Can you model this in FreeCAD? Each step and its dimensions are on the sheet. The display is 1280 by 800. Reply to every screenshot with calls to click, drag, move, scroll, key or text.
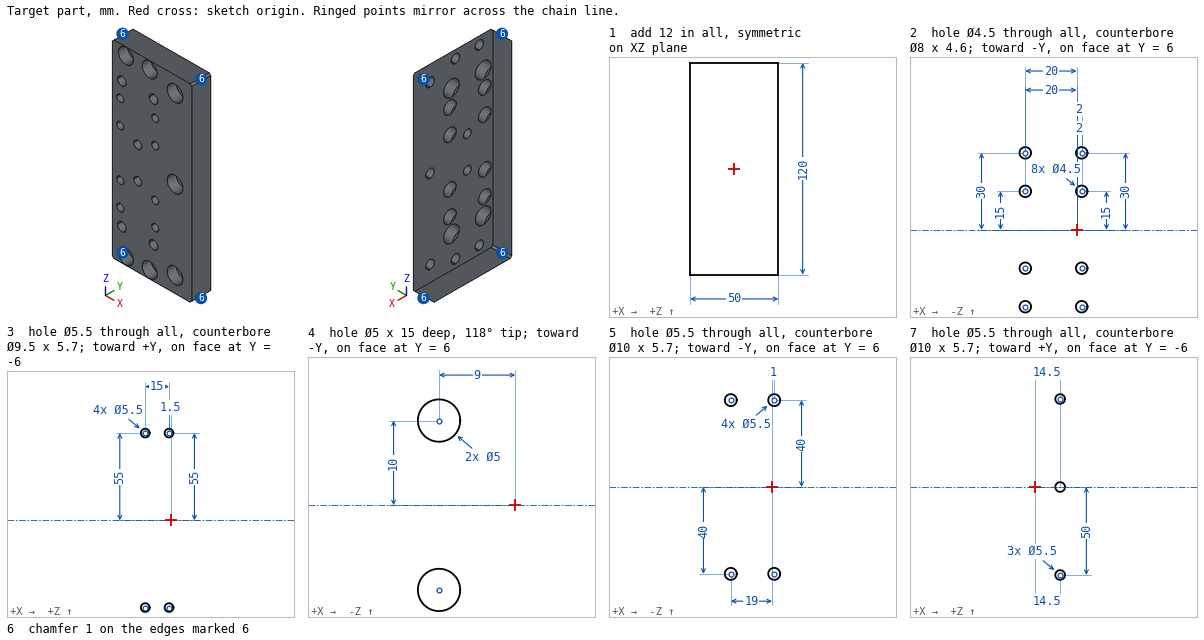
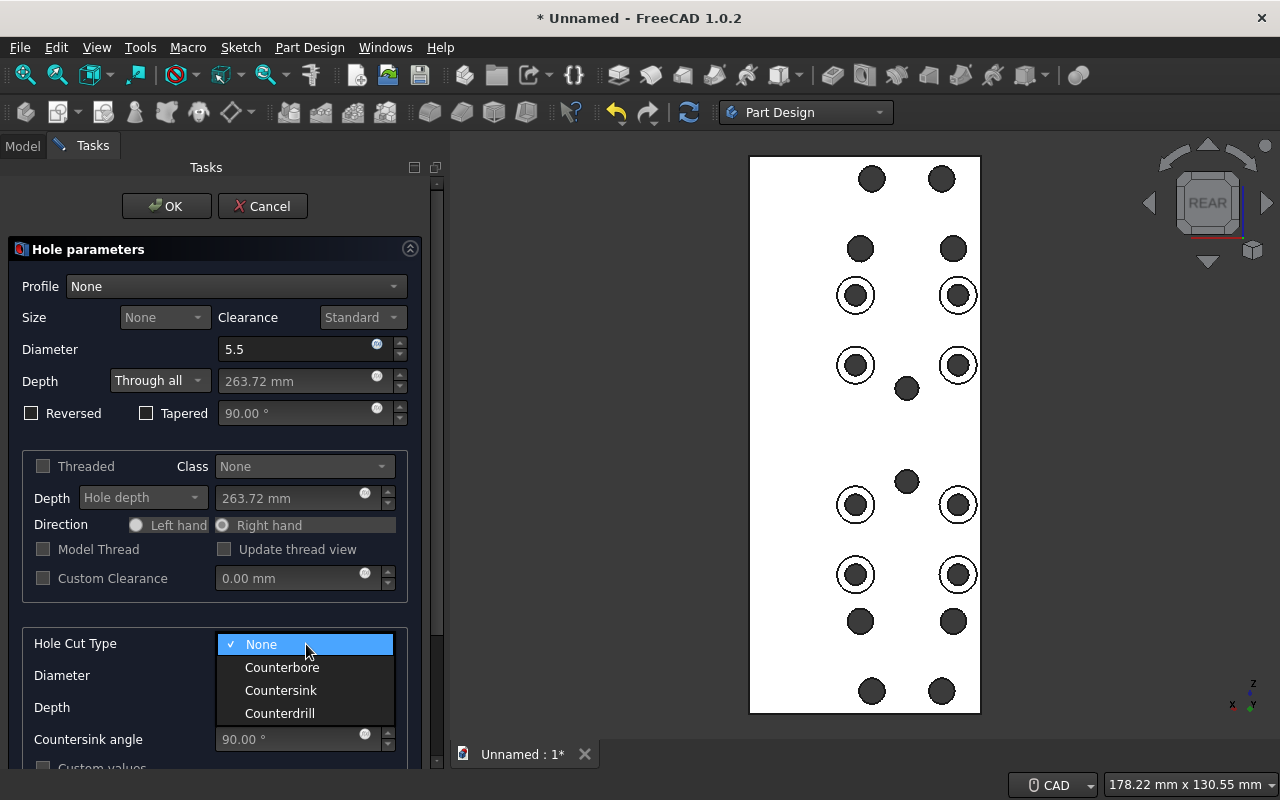
click(304, 668)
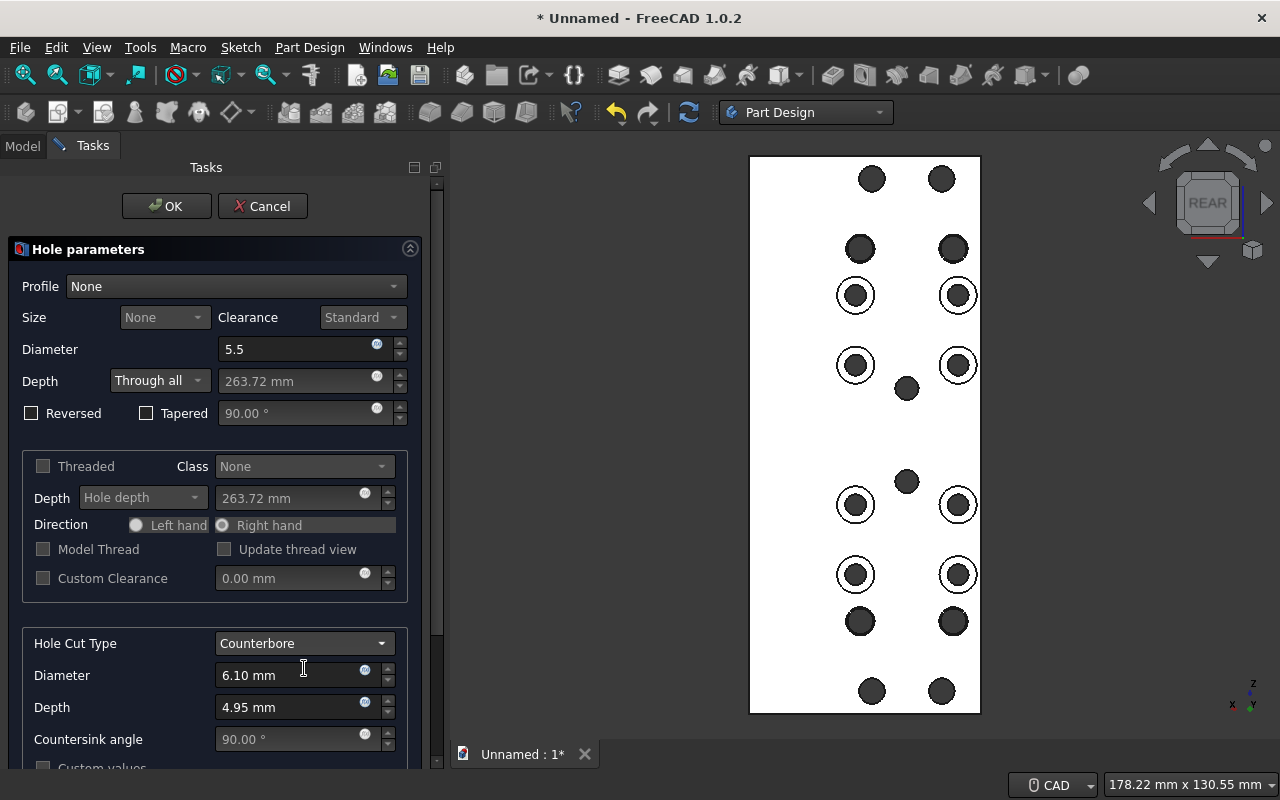
triple_click(298, 675)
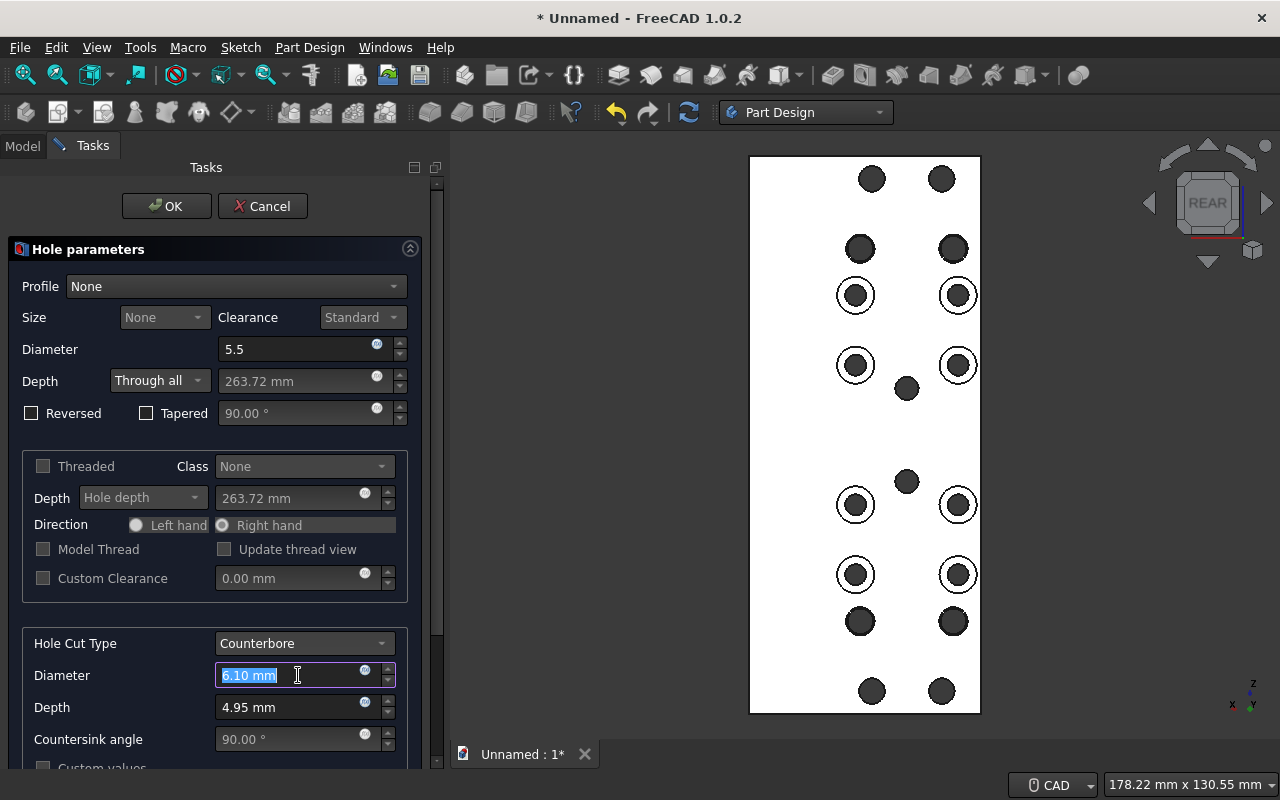
text(10)
key(Tab)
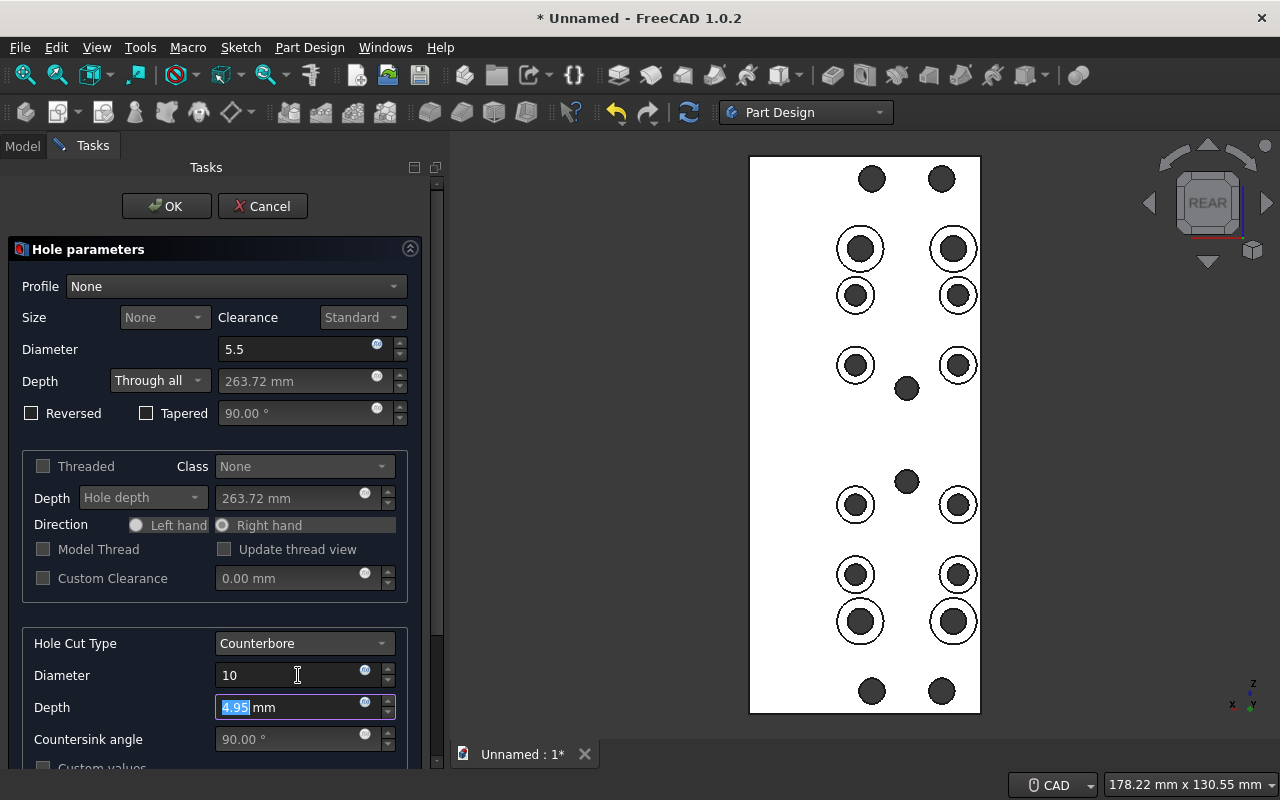
text(5.7)
key(Tab)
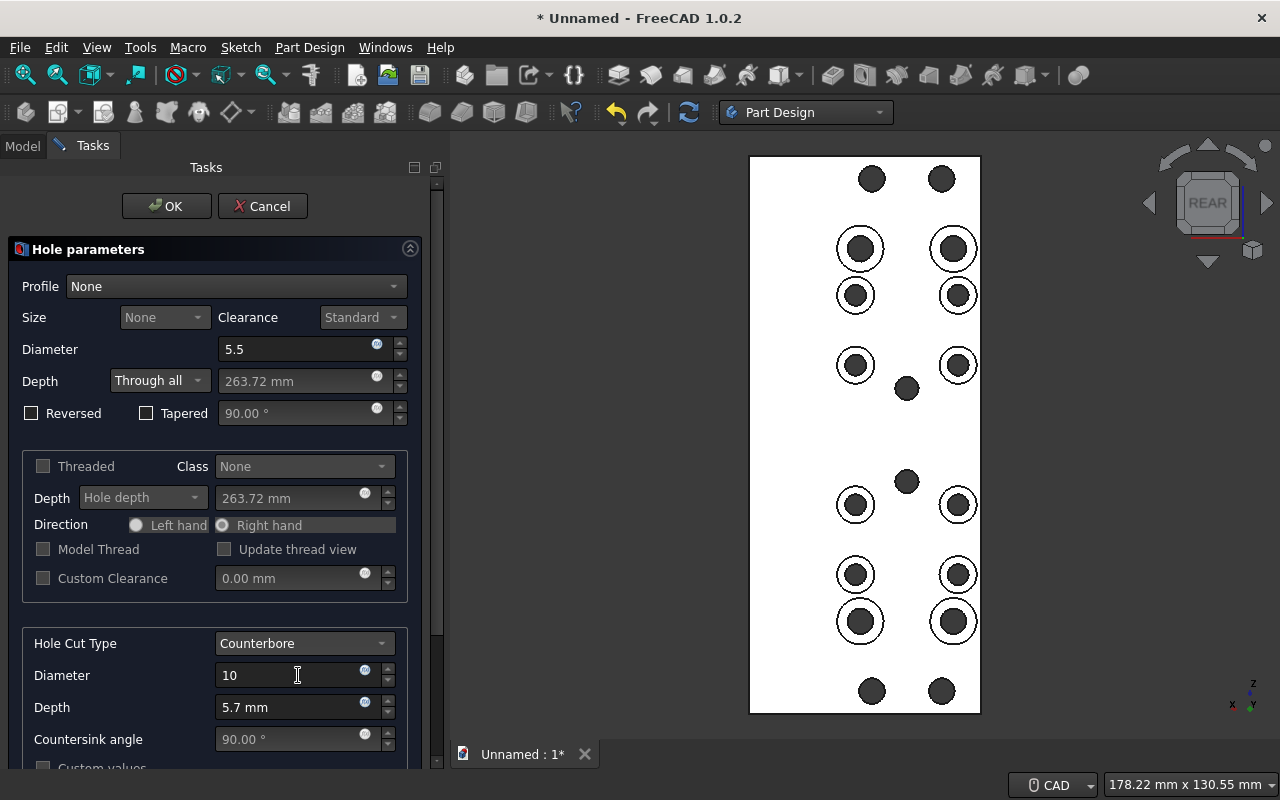
click(167, 206)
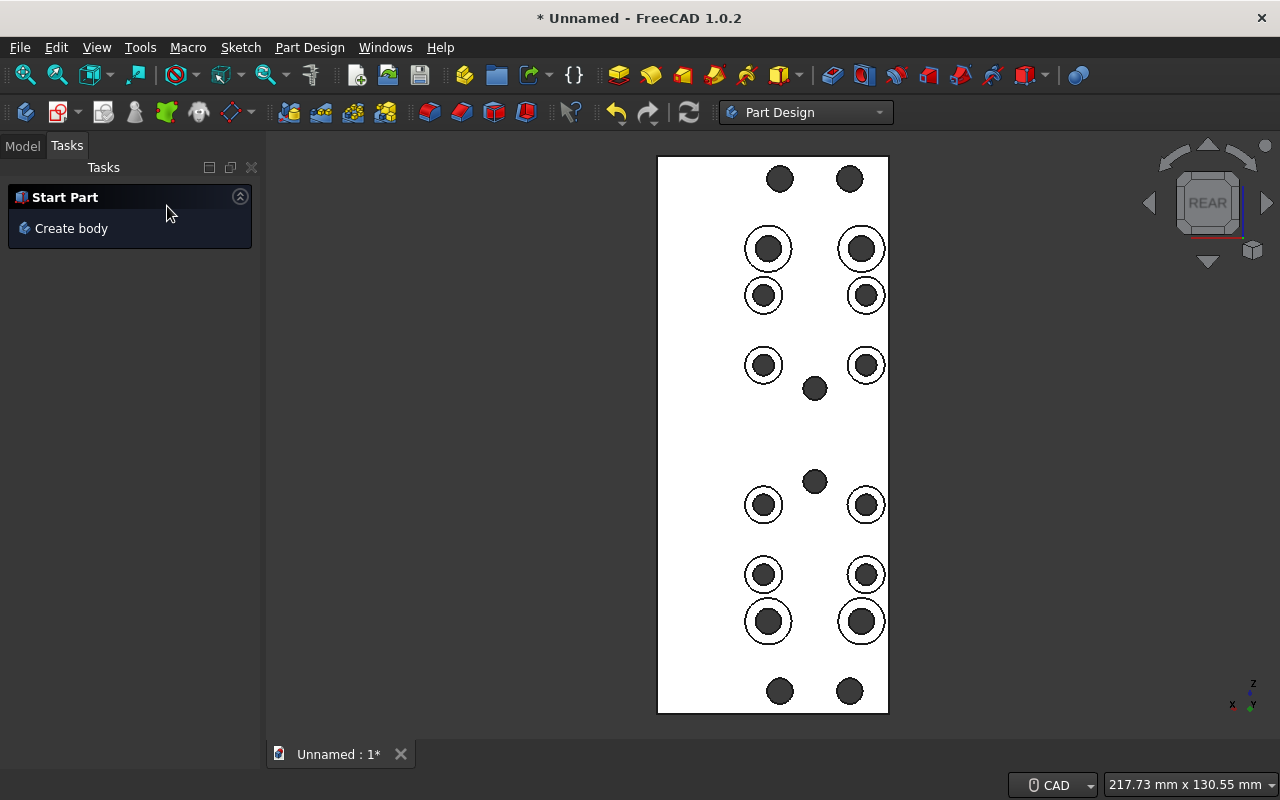
key(0)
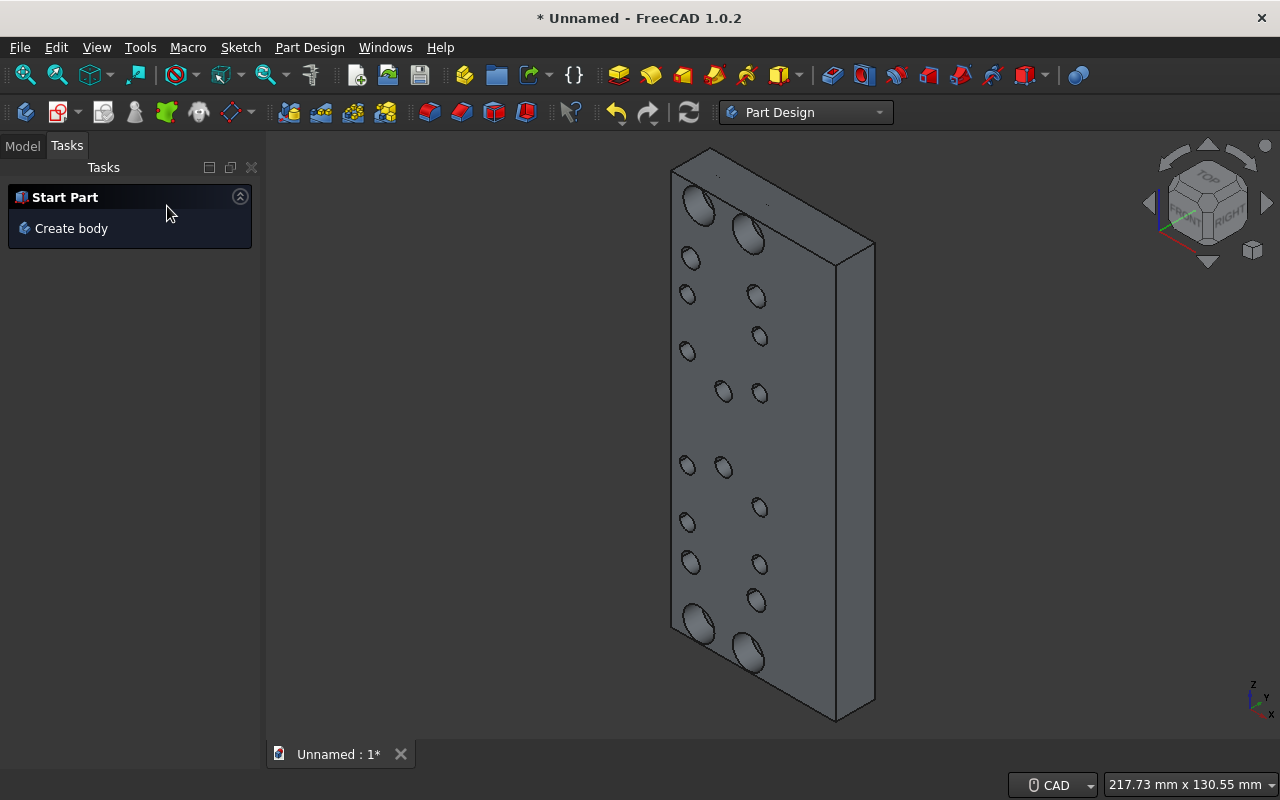
click(855, 253)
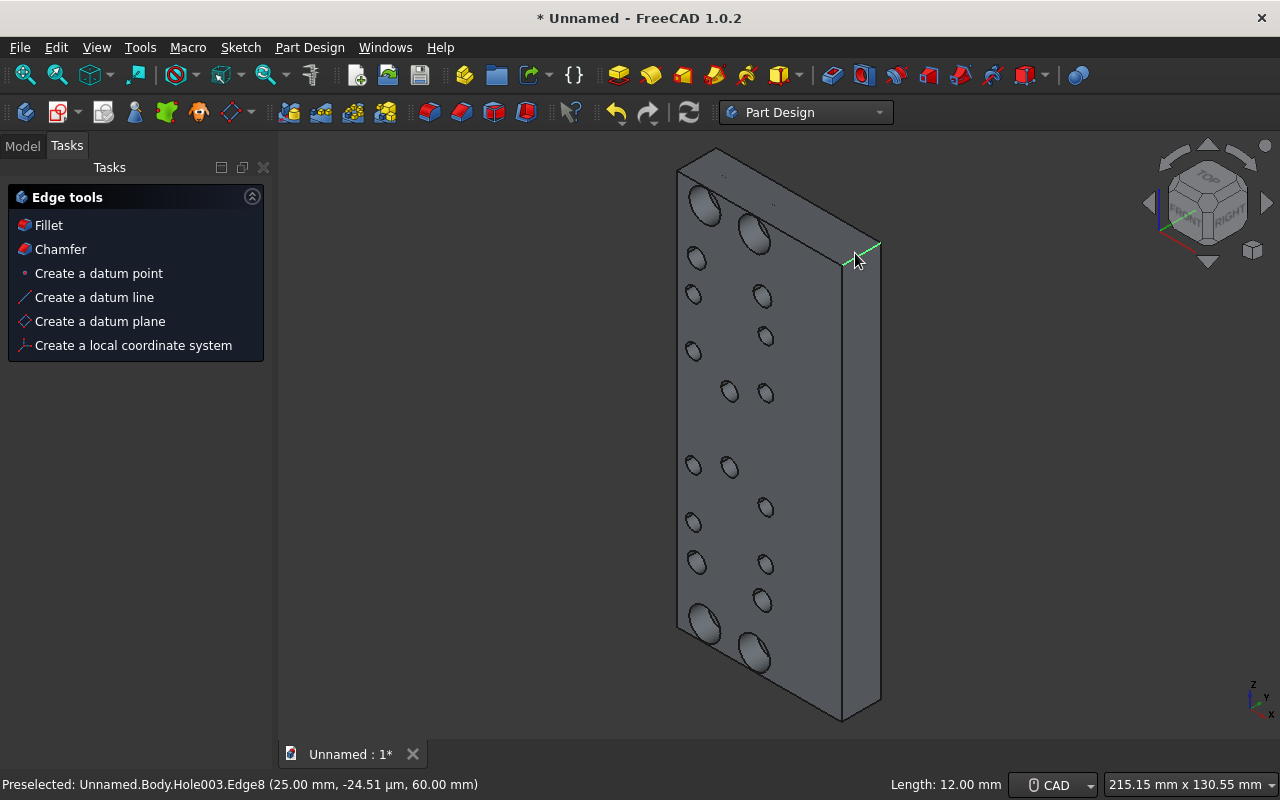
key(2)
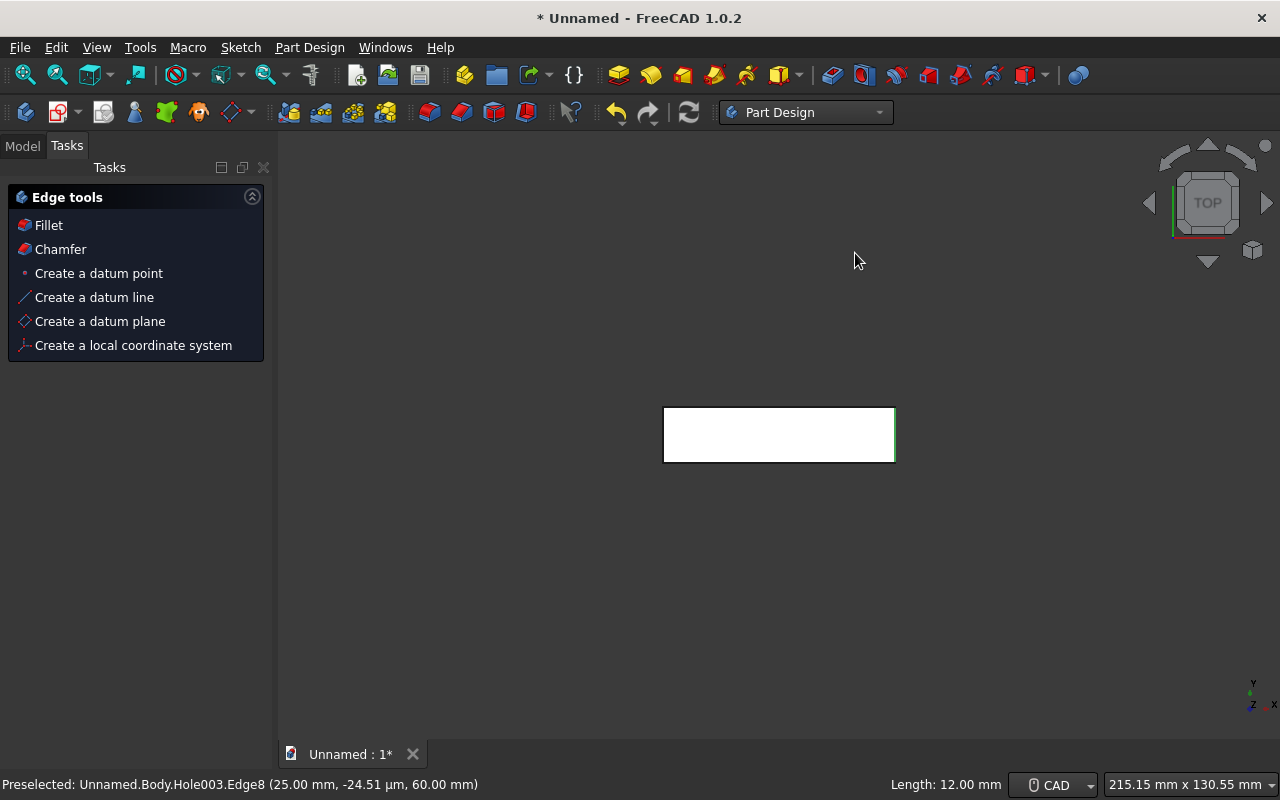
click(26, 76)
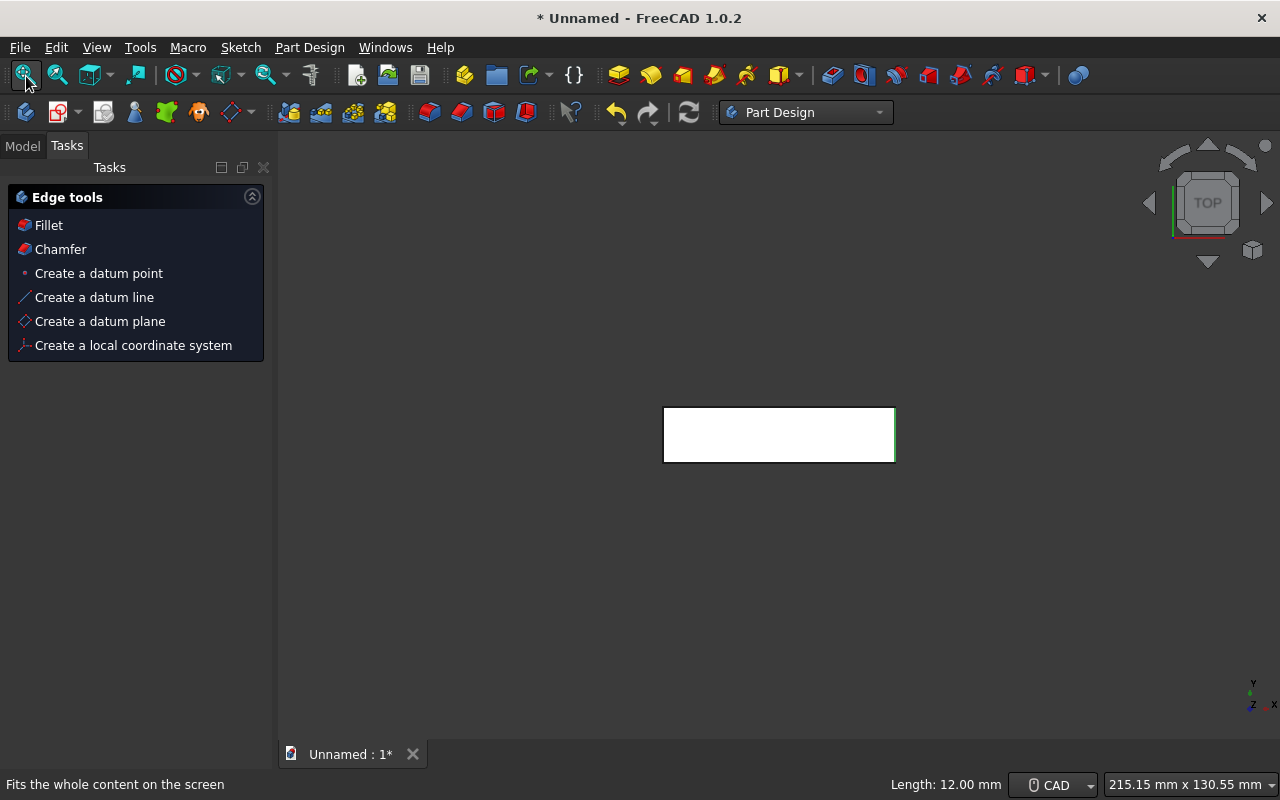
click(663, 434, ctrl)